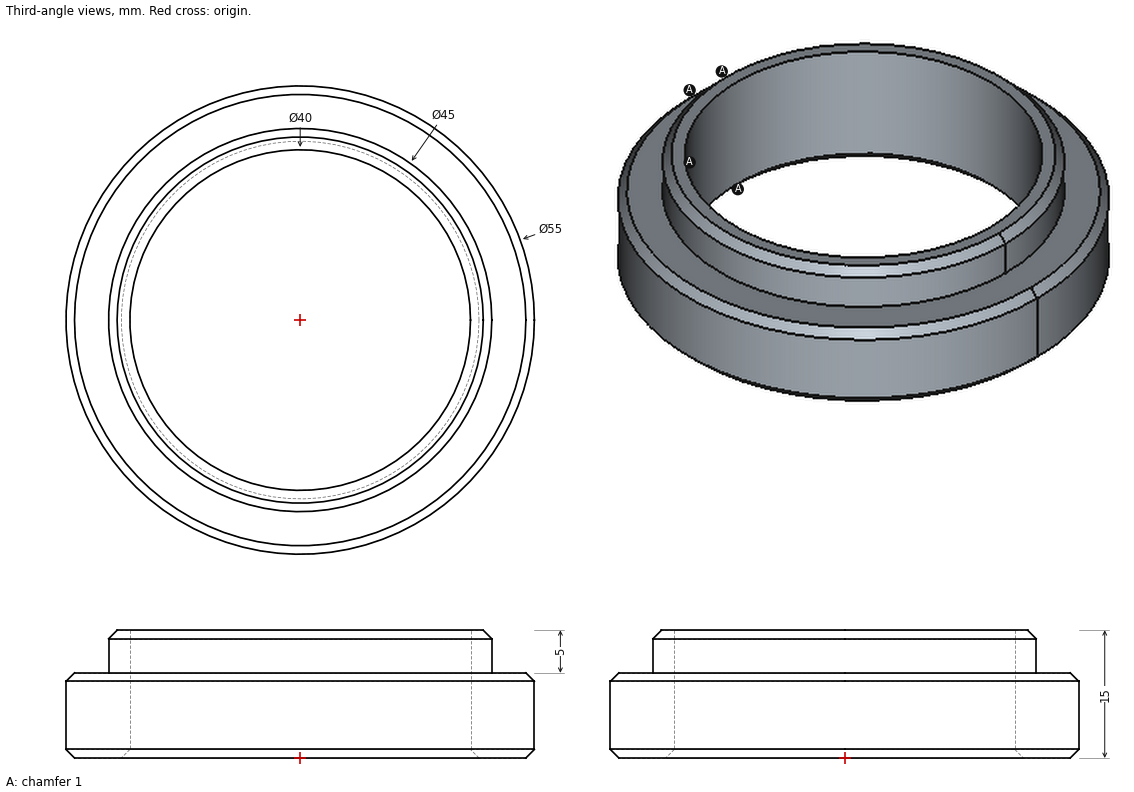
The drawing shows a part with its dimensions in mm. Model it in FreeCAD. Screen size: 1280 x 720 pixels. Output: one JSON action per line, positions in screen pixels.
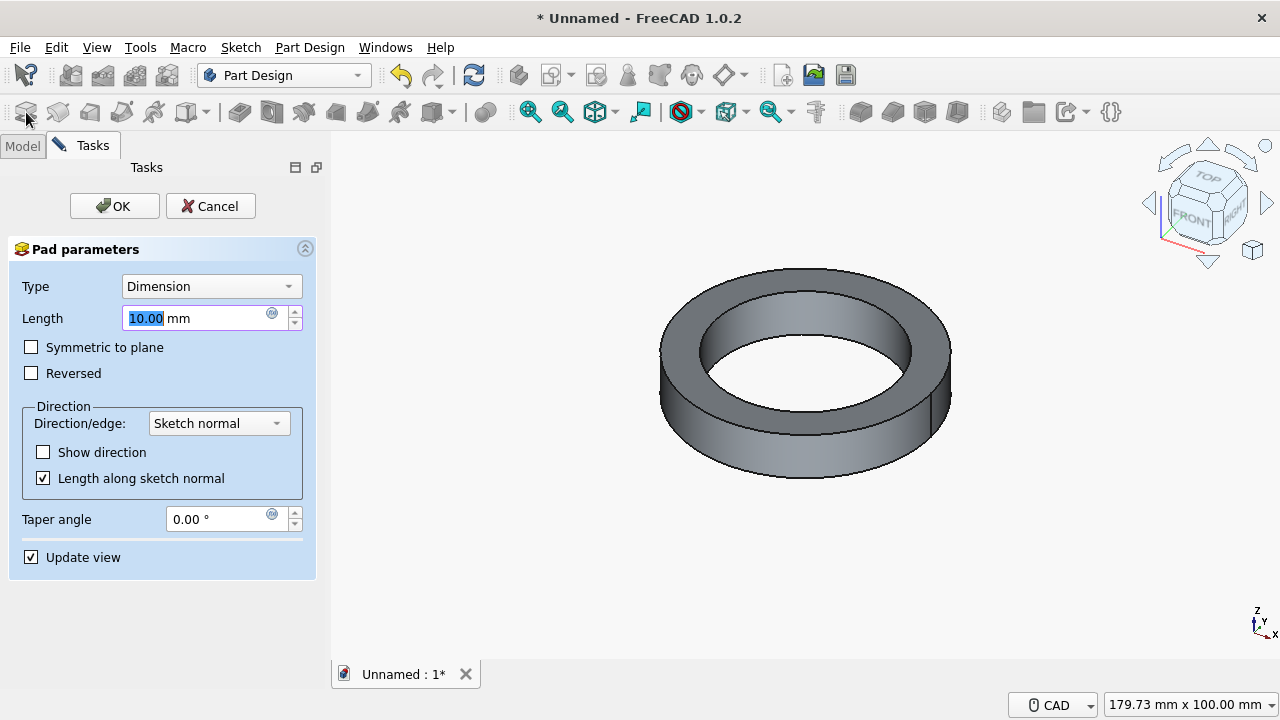
{"action": "type", "text": "15"}
{"action": "key", "text": "Tab"}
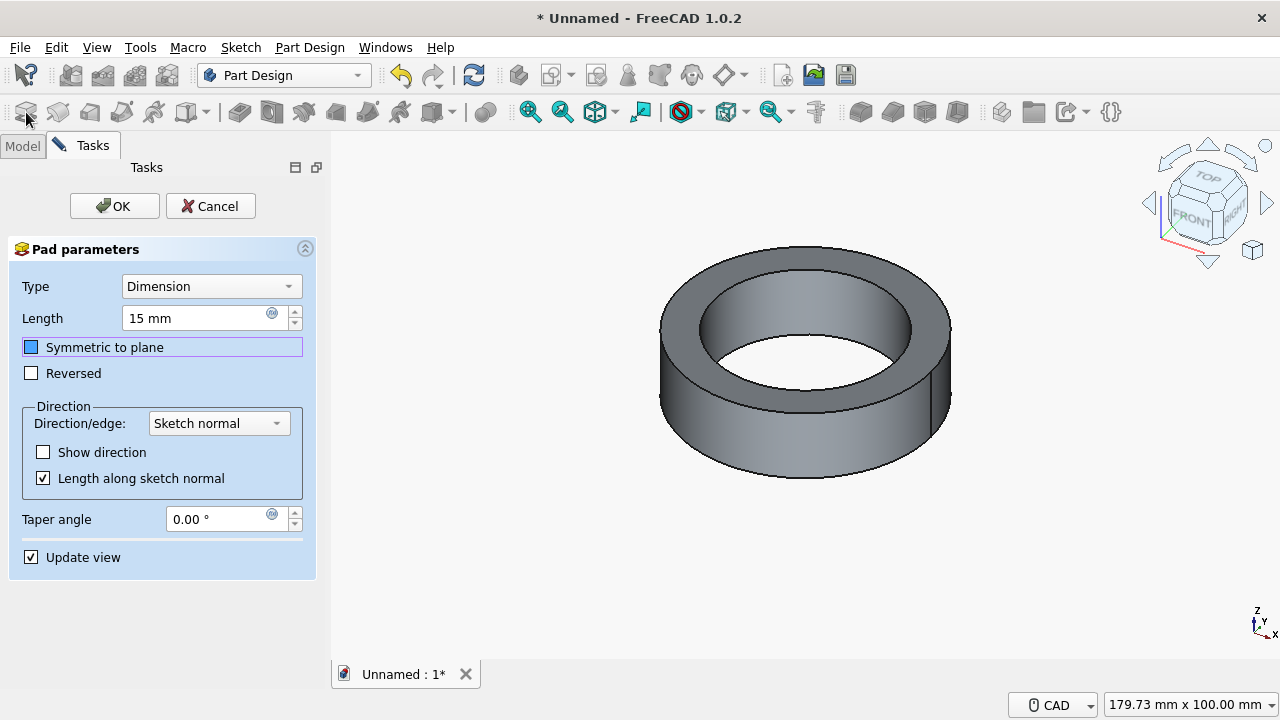
{"action": "left_click", "coordinate": [115, 206]}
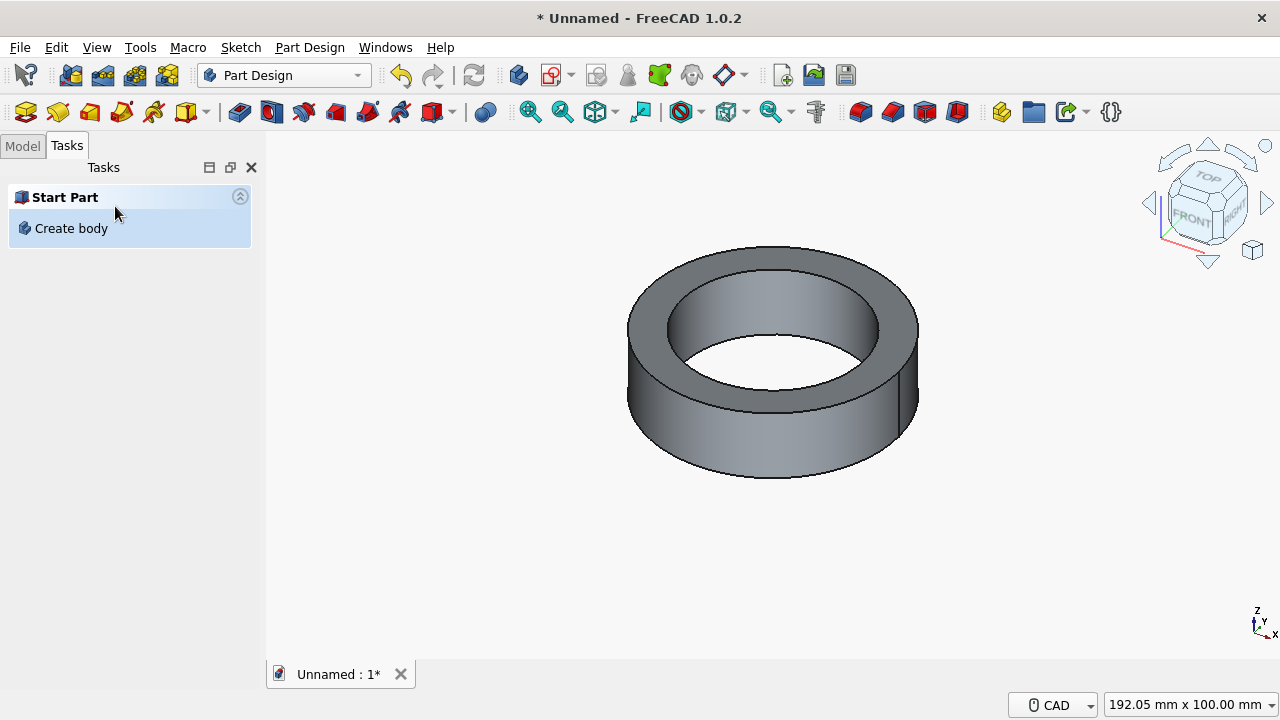
{"action": "left_click", "coordinate": [23, 145]}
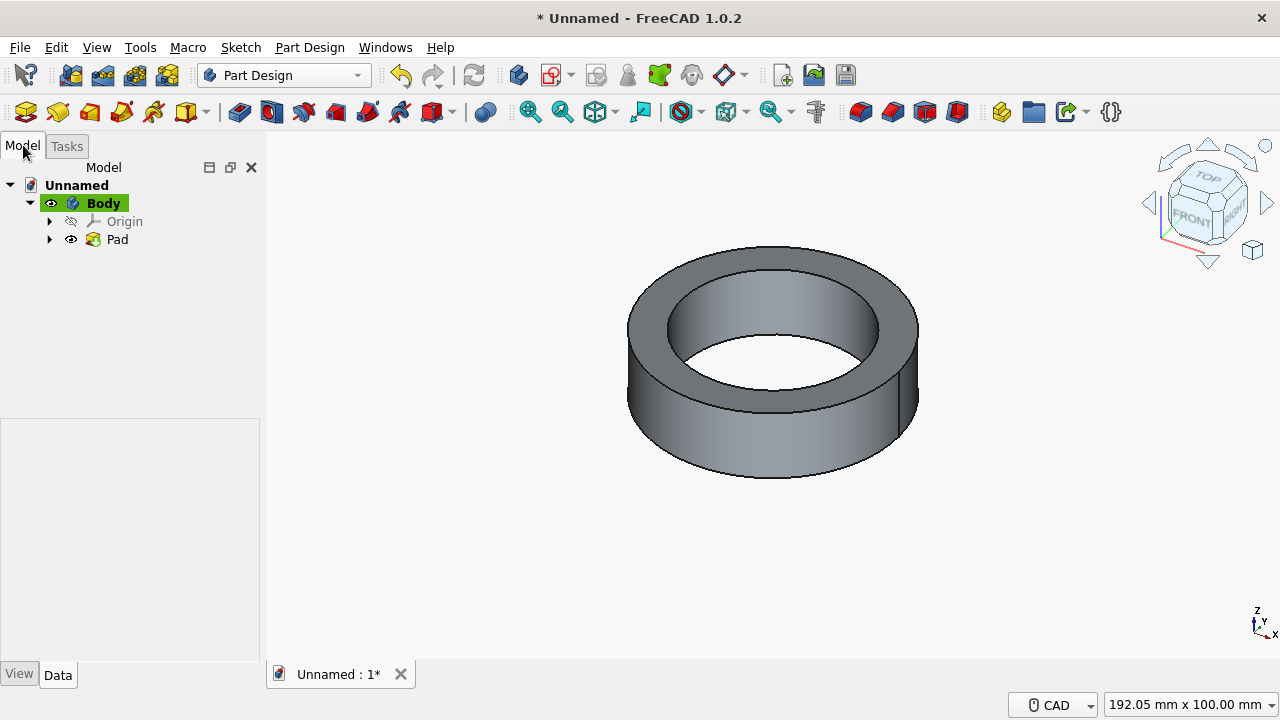
{"action": "left_click", "coordinate": [50, 221]}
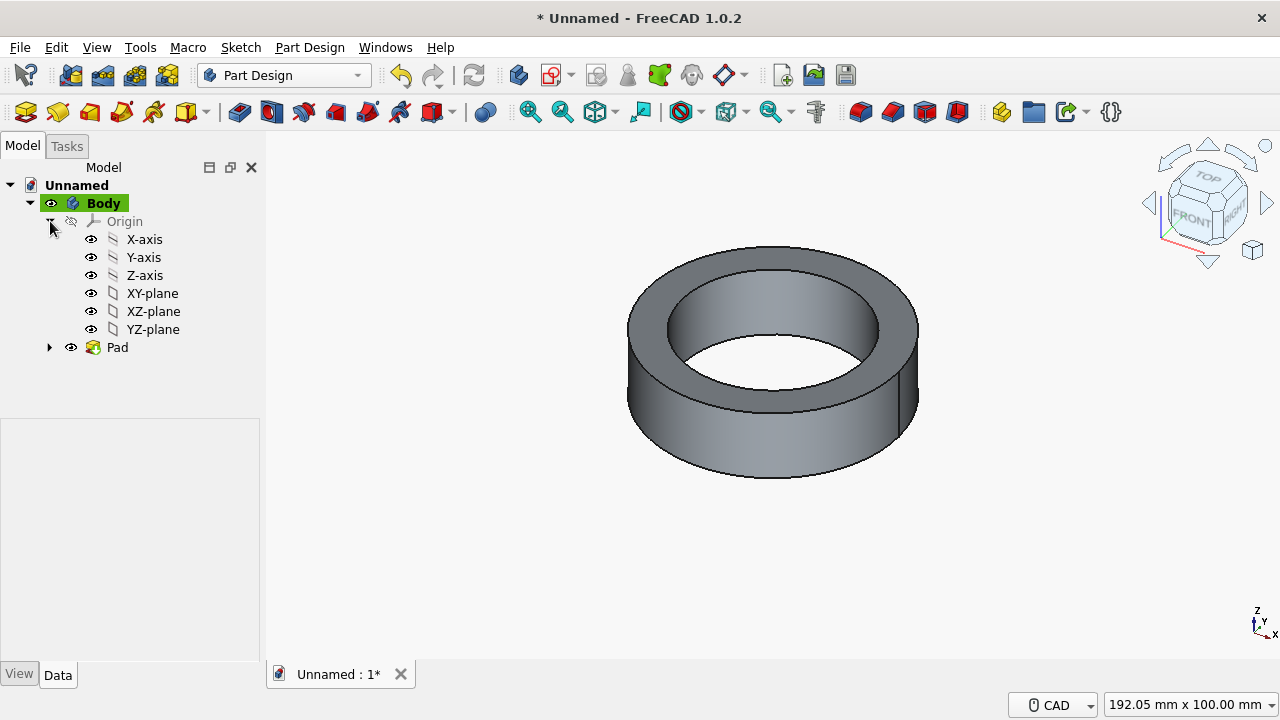
{"action": "left_click", "coordinate": [136, 293]}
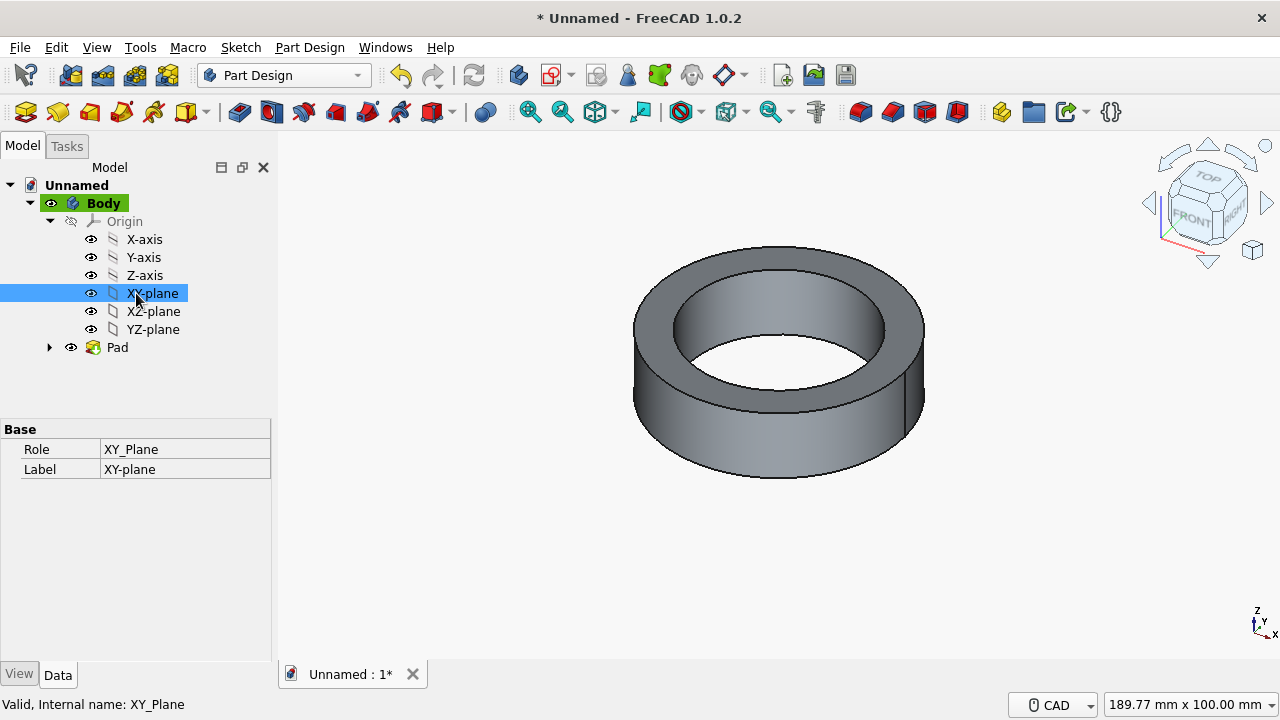
{"action": "left_click", "coordinate": [724, 76]}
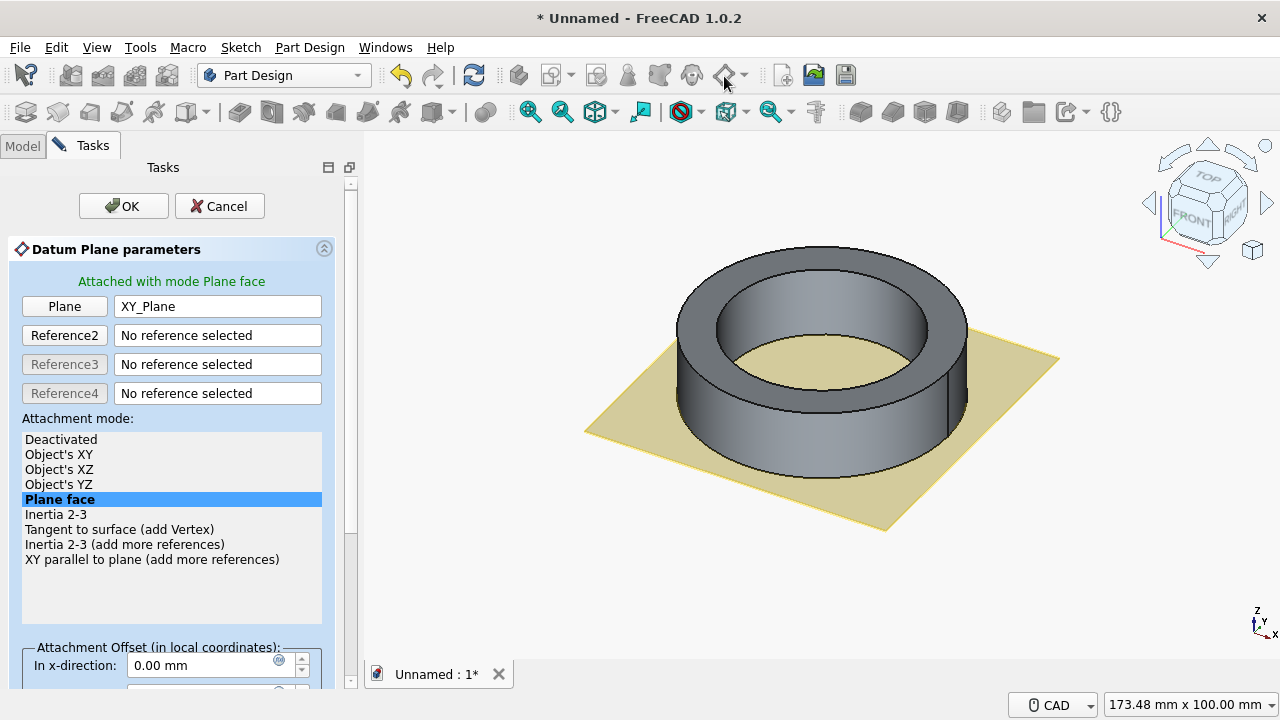
{"action": "scroll", "coordinate": [351, 432], "scroll_direction": "down", "scroll_amount": 2}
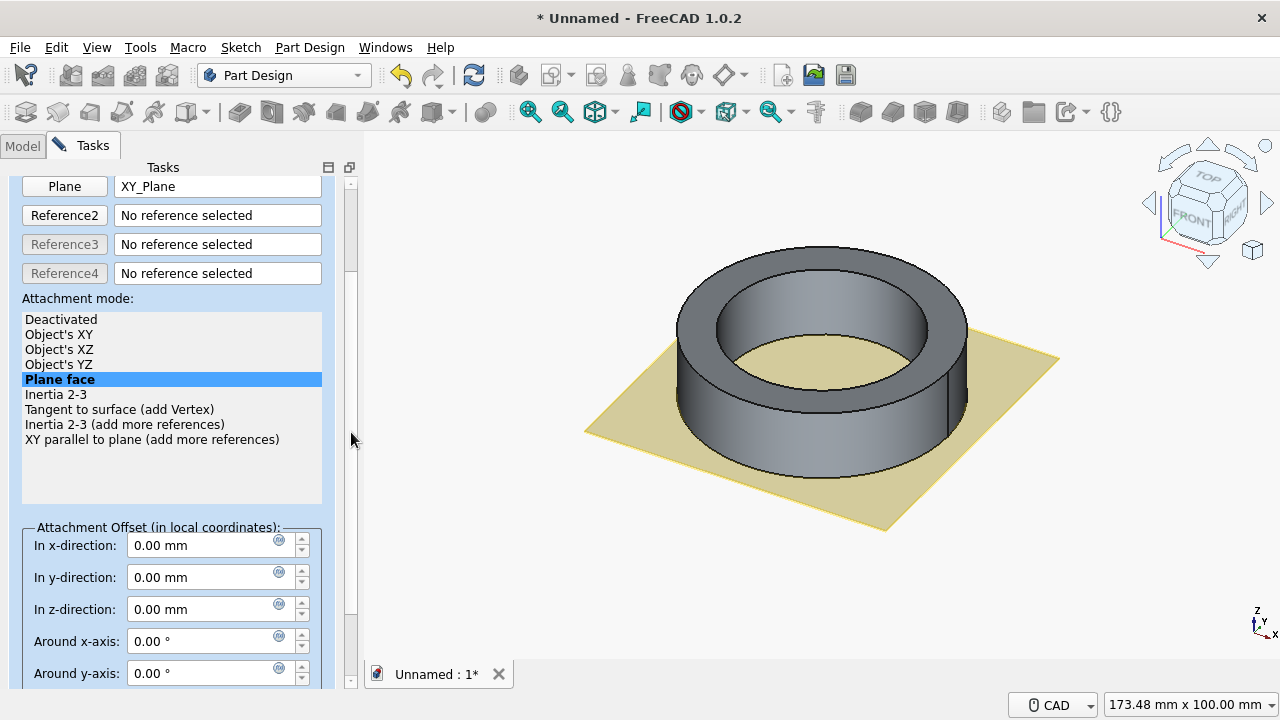
{"action": "triple_click", "coordinate": [210, 609]}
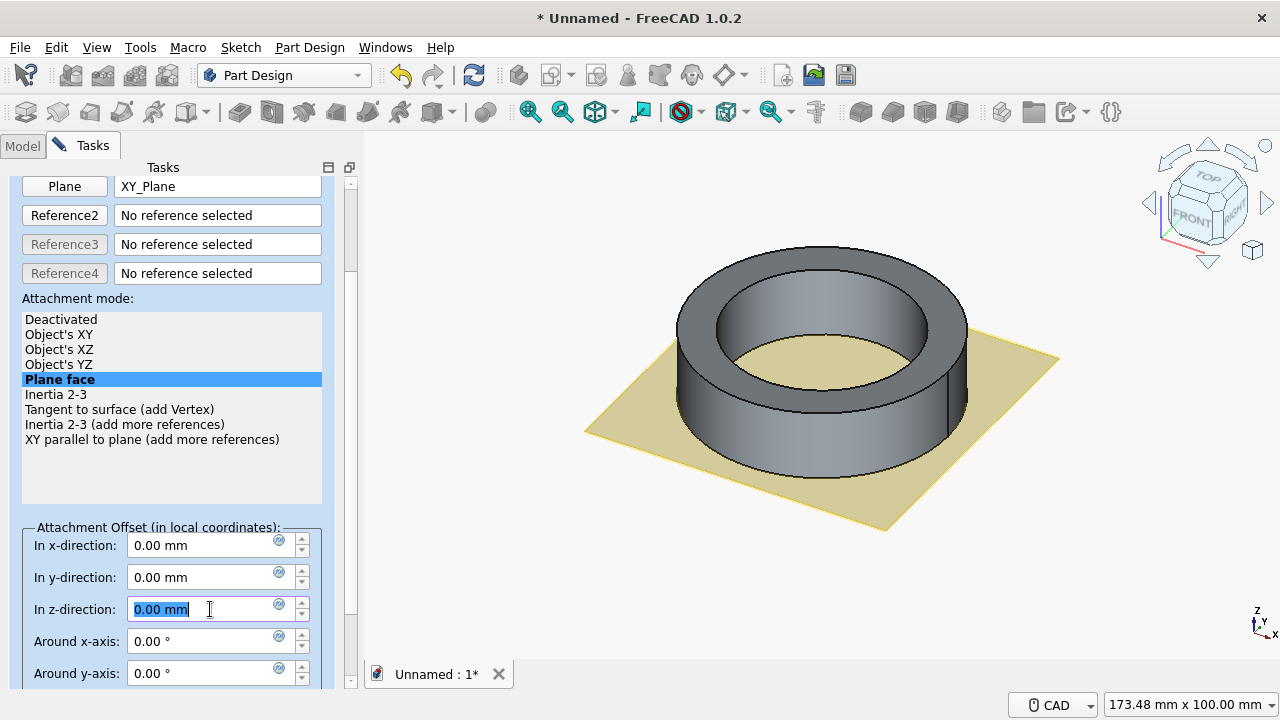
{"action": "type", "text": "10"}
{"action": "key", "text": "Tab"}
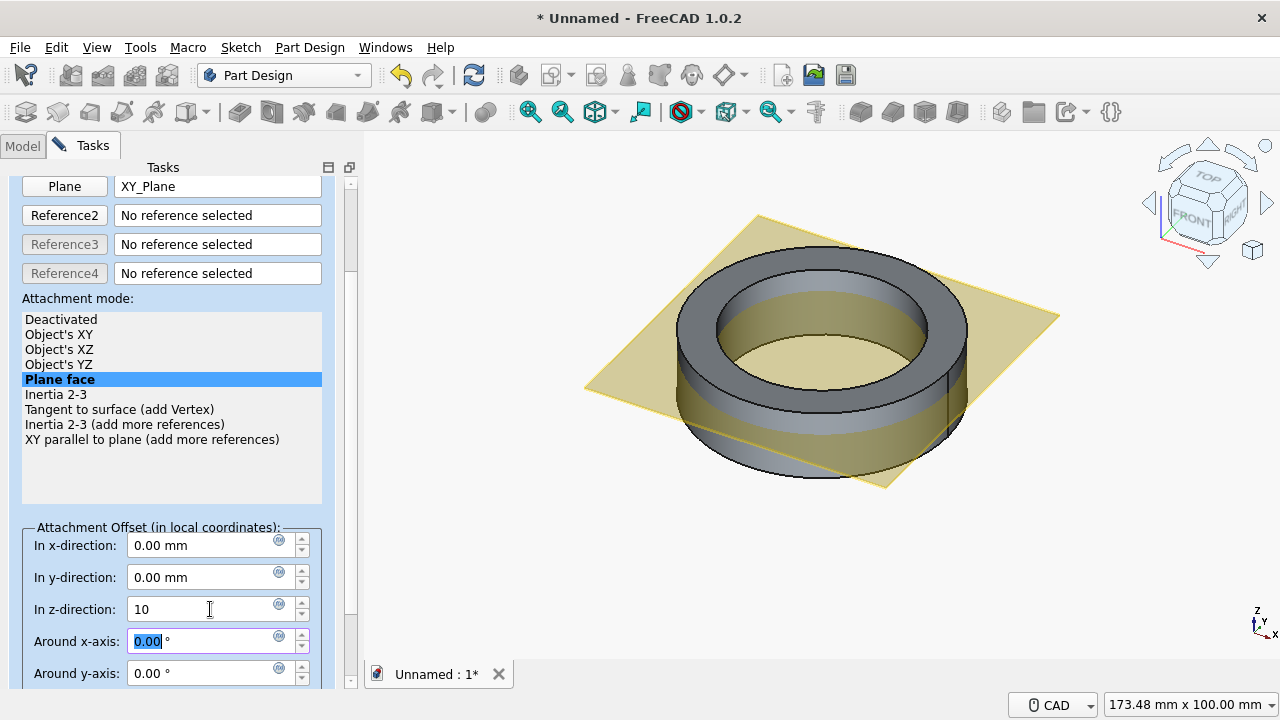
{"action": "scroll", "coordinate": [351, 432], "scroll_direction": "up", "scroll_amount": 3}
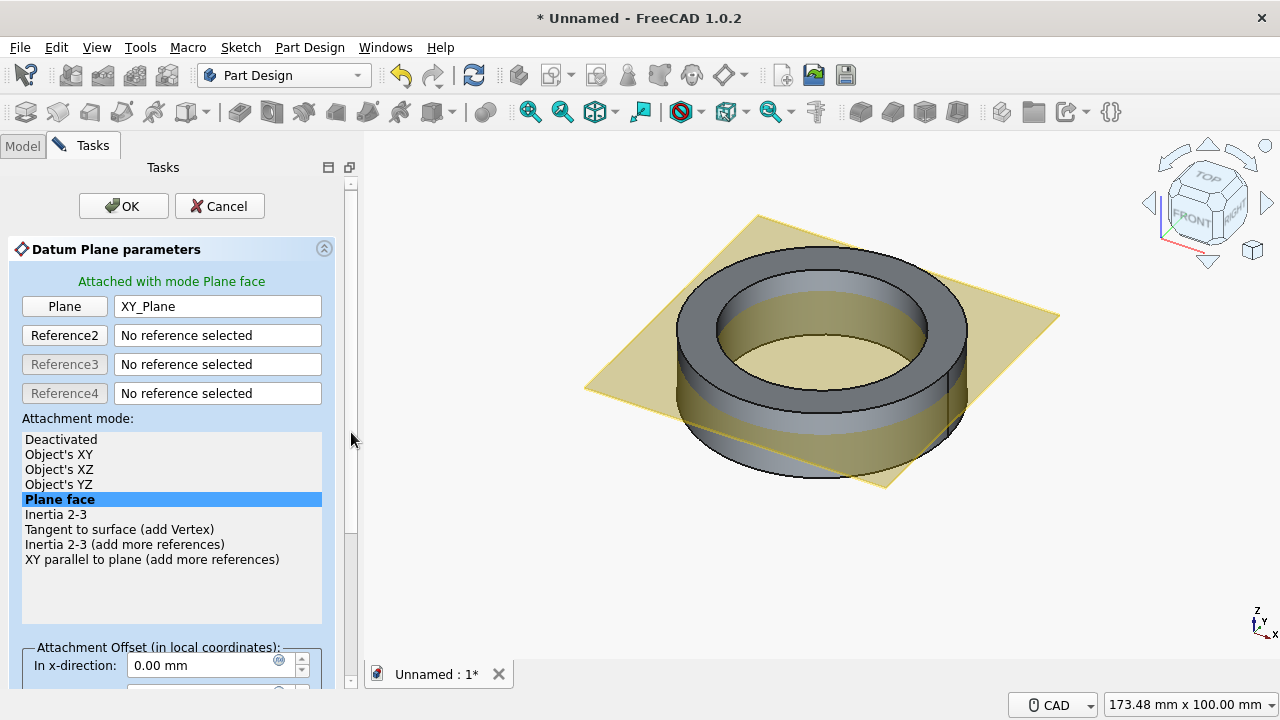
{"action": "left_click", "coordinate": [124, 206]}